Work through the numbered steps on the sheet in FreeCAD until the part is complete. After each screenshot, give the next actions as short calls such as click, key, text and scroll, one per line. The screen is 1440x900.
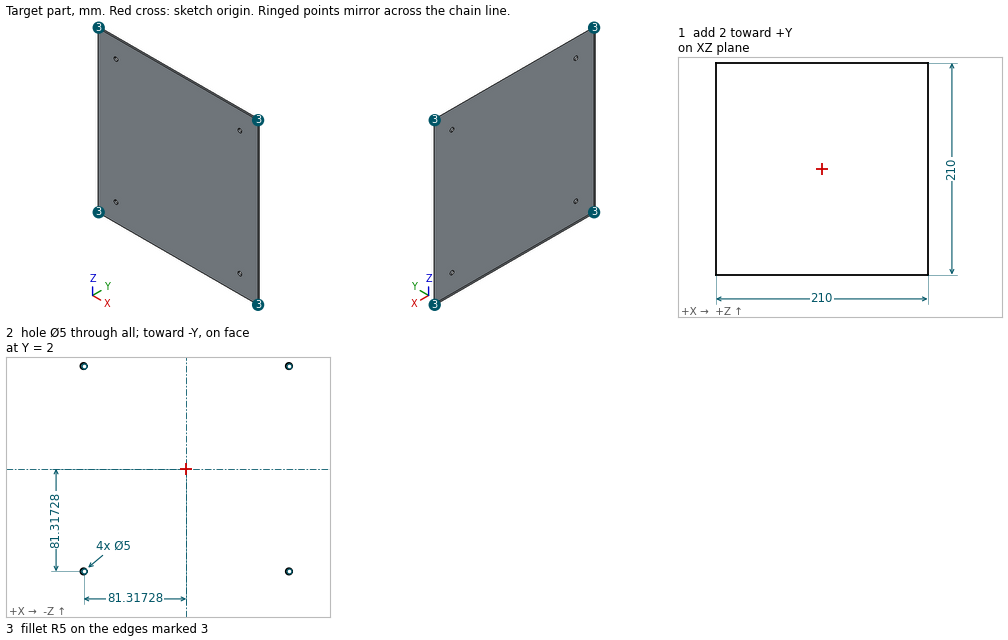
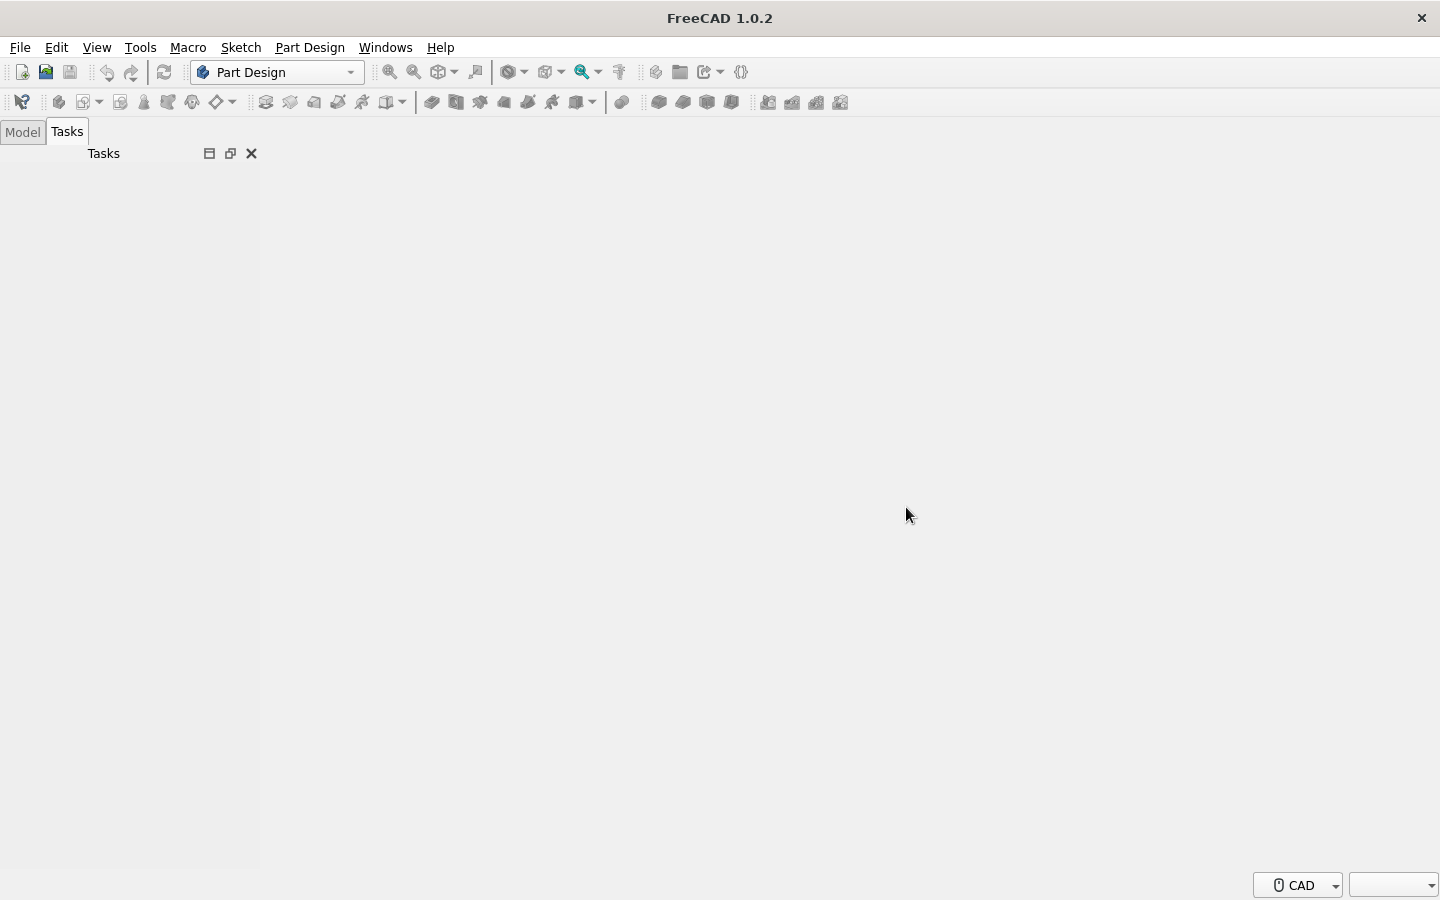
click(22, 72)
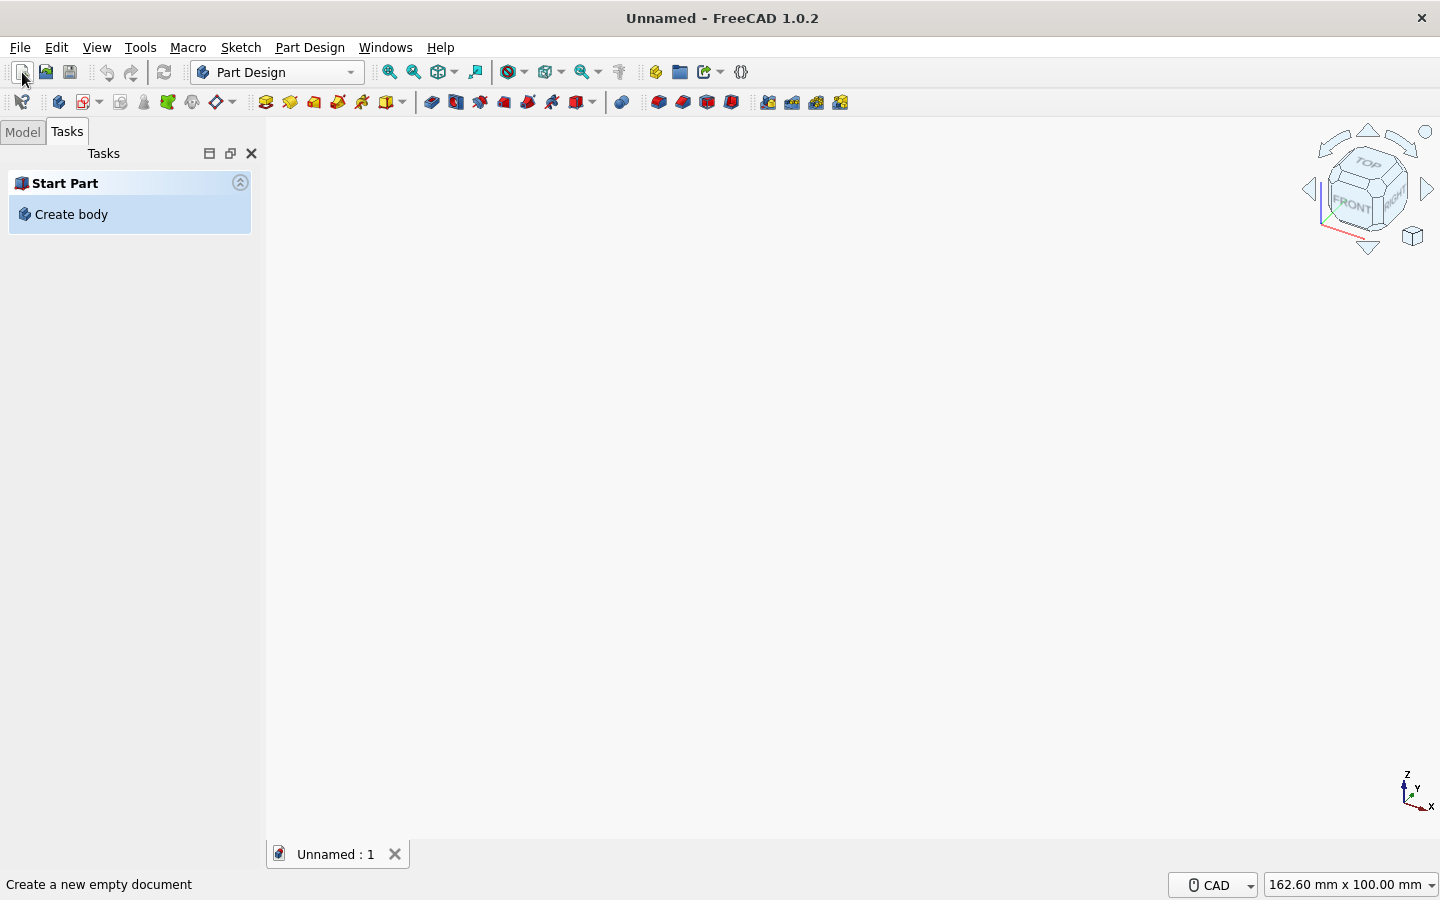
click(84, 102)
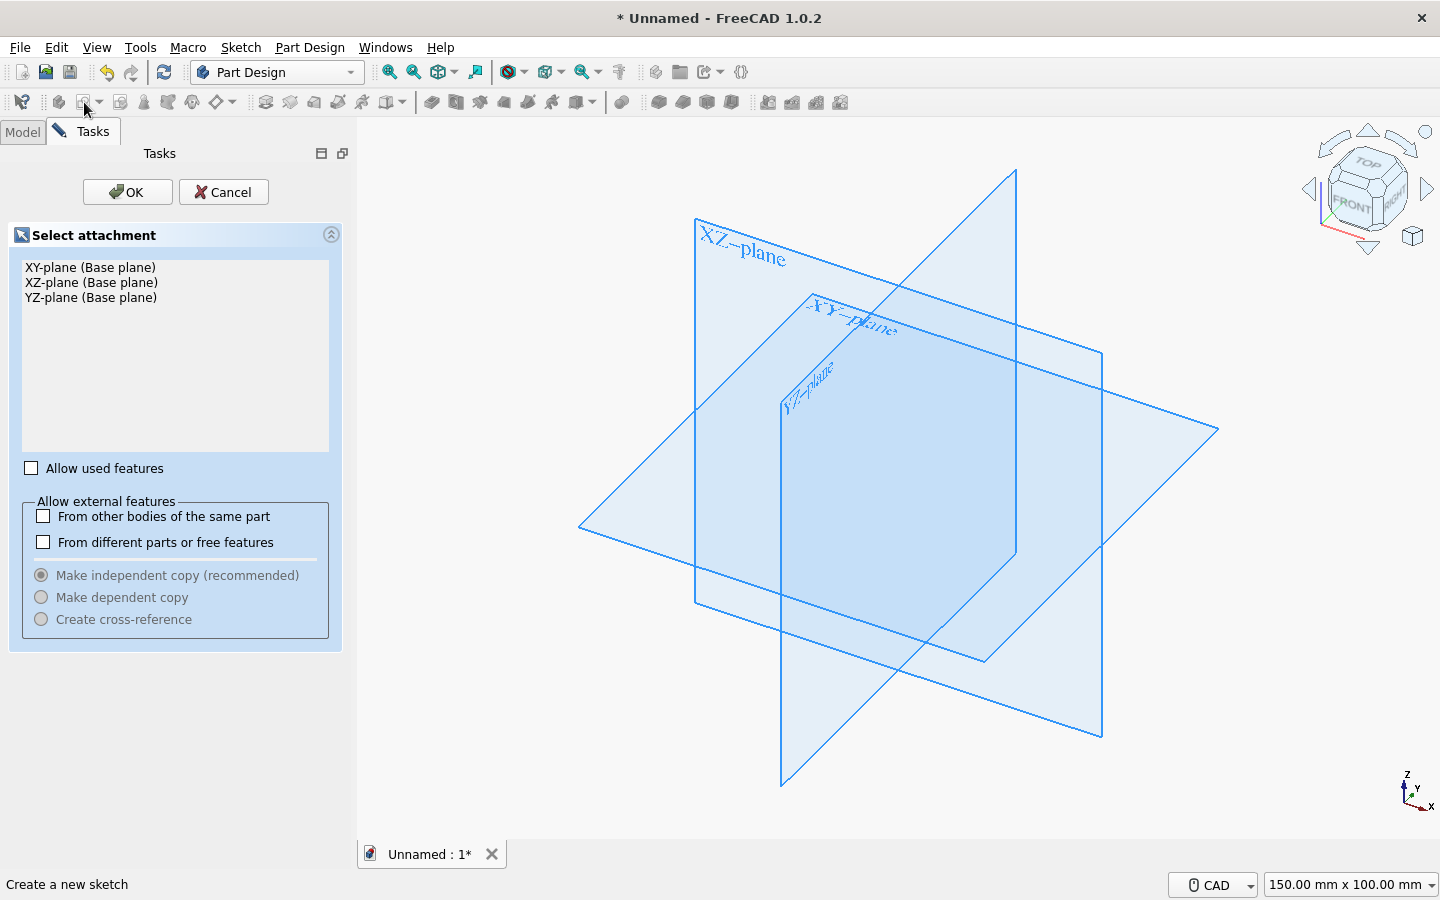
click(82, 282)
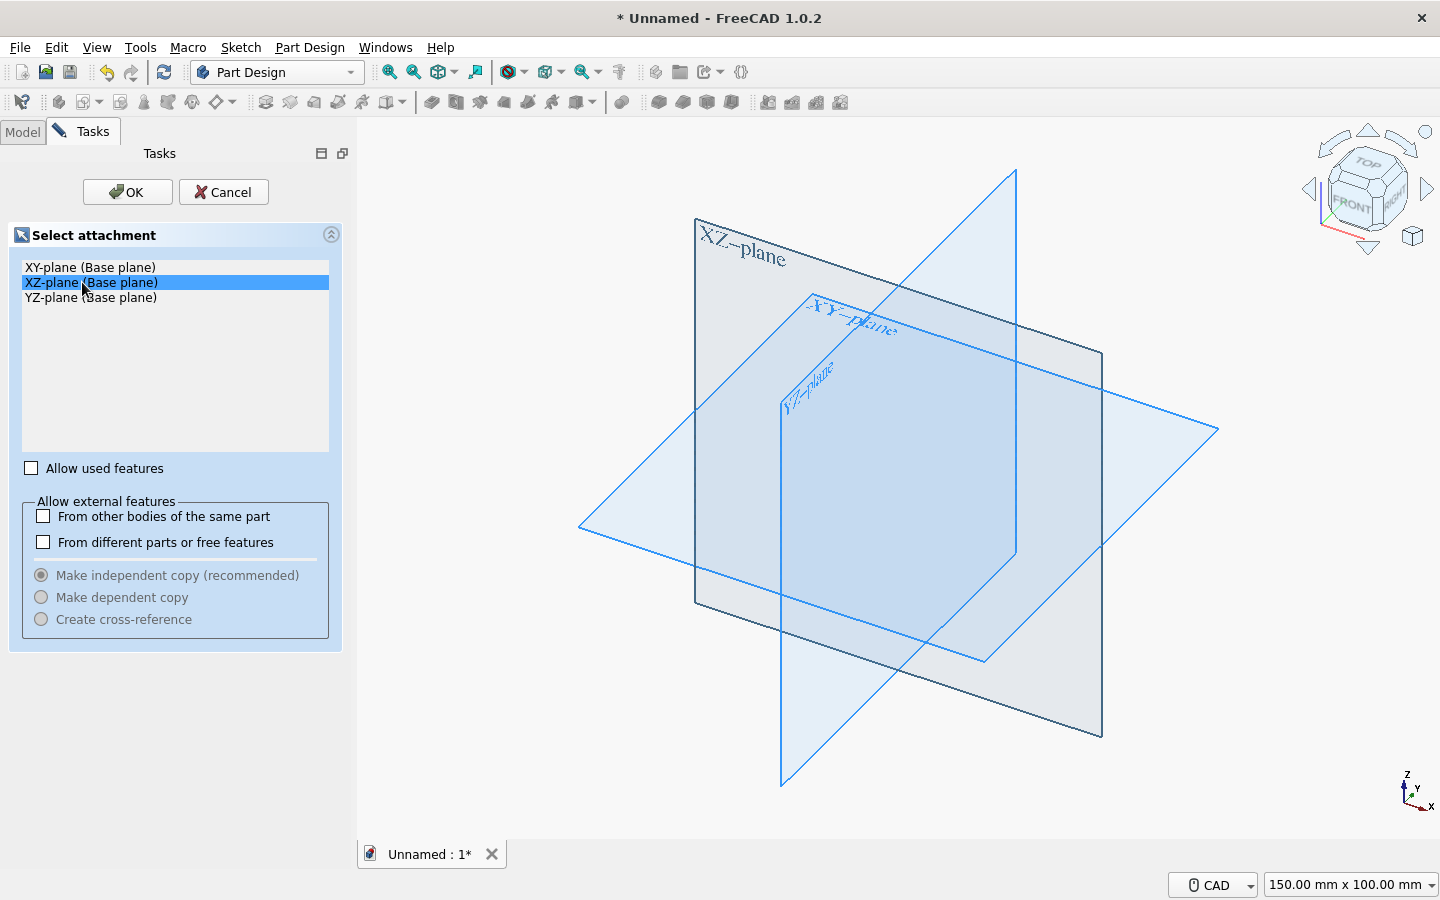
click(128, 192)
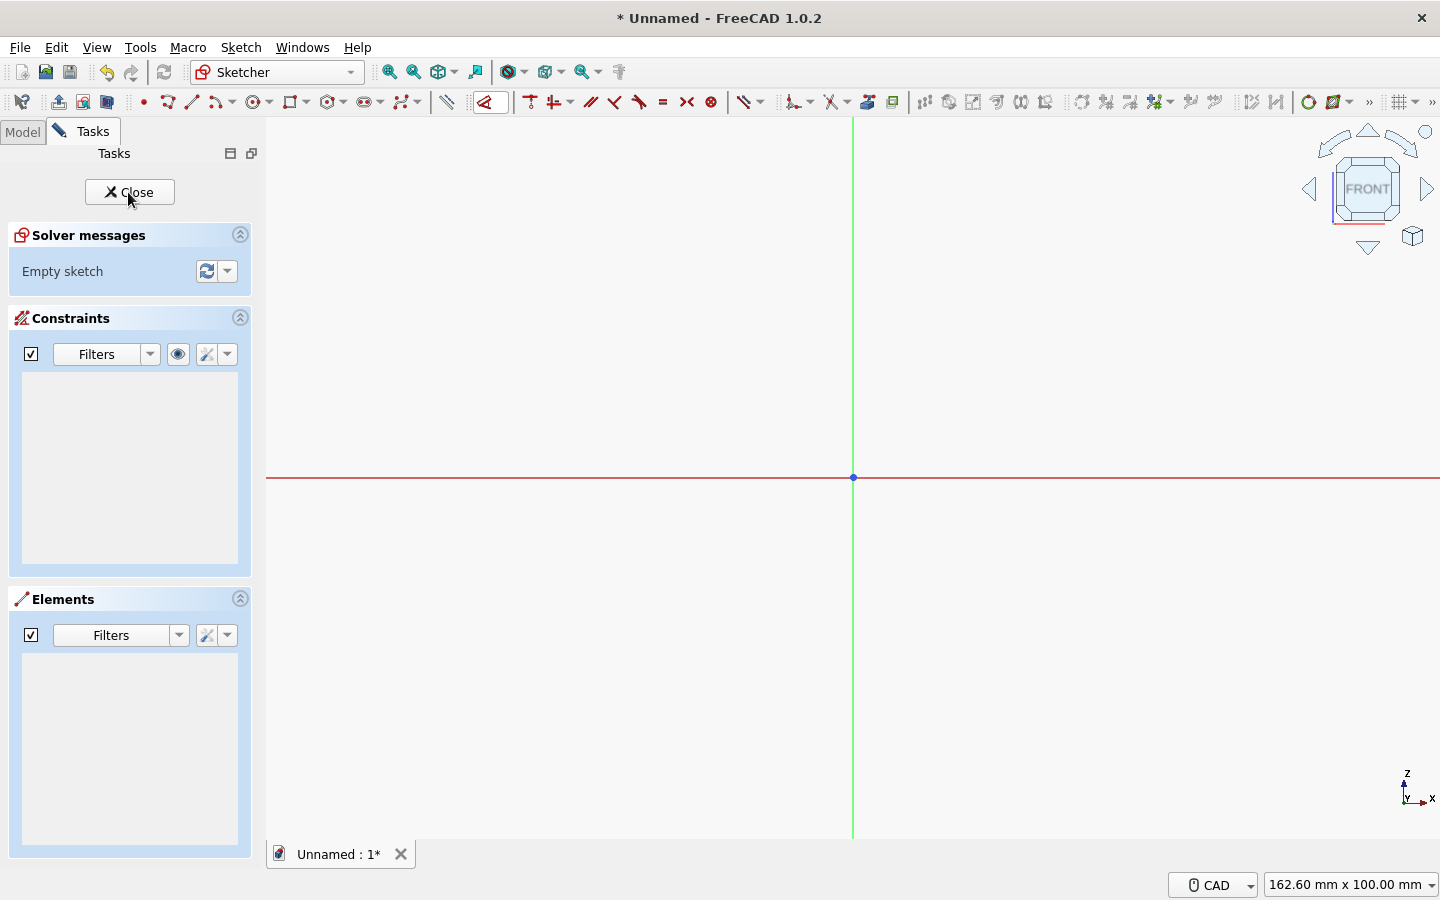
scroll(755, 478, down, 6)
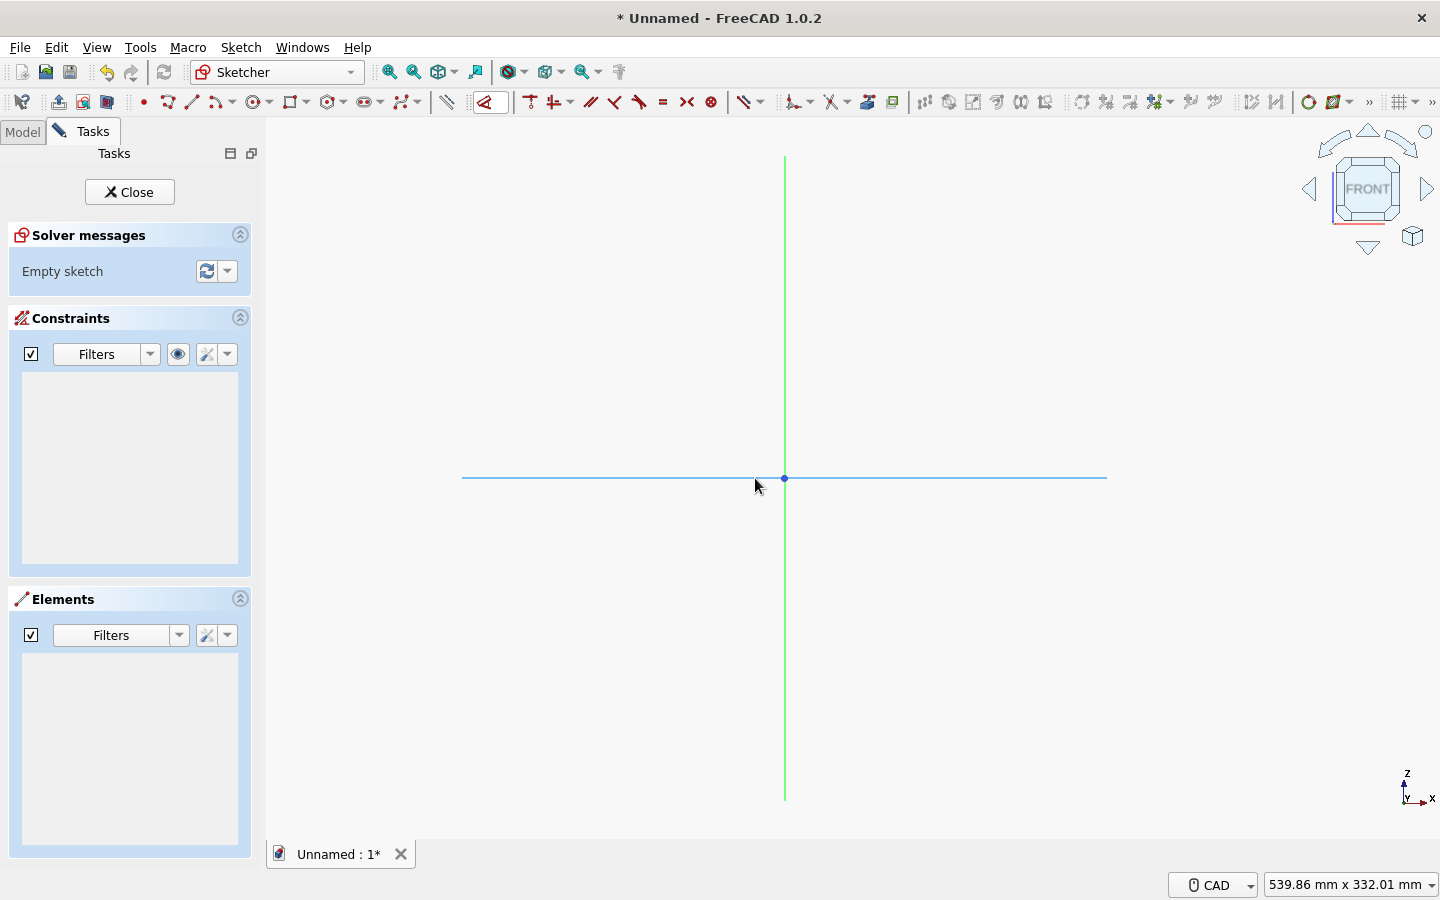
key(g)
key(v)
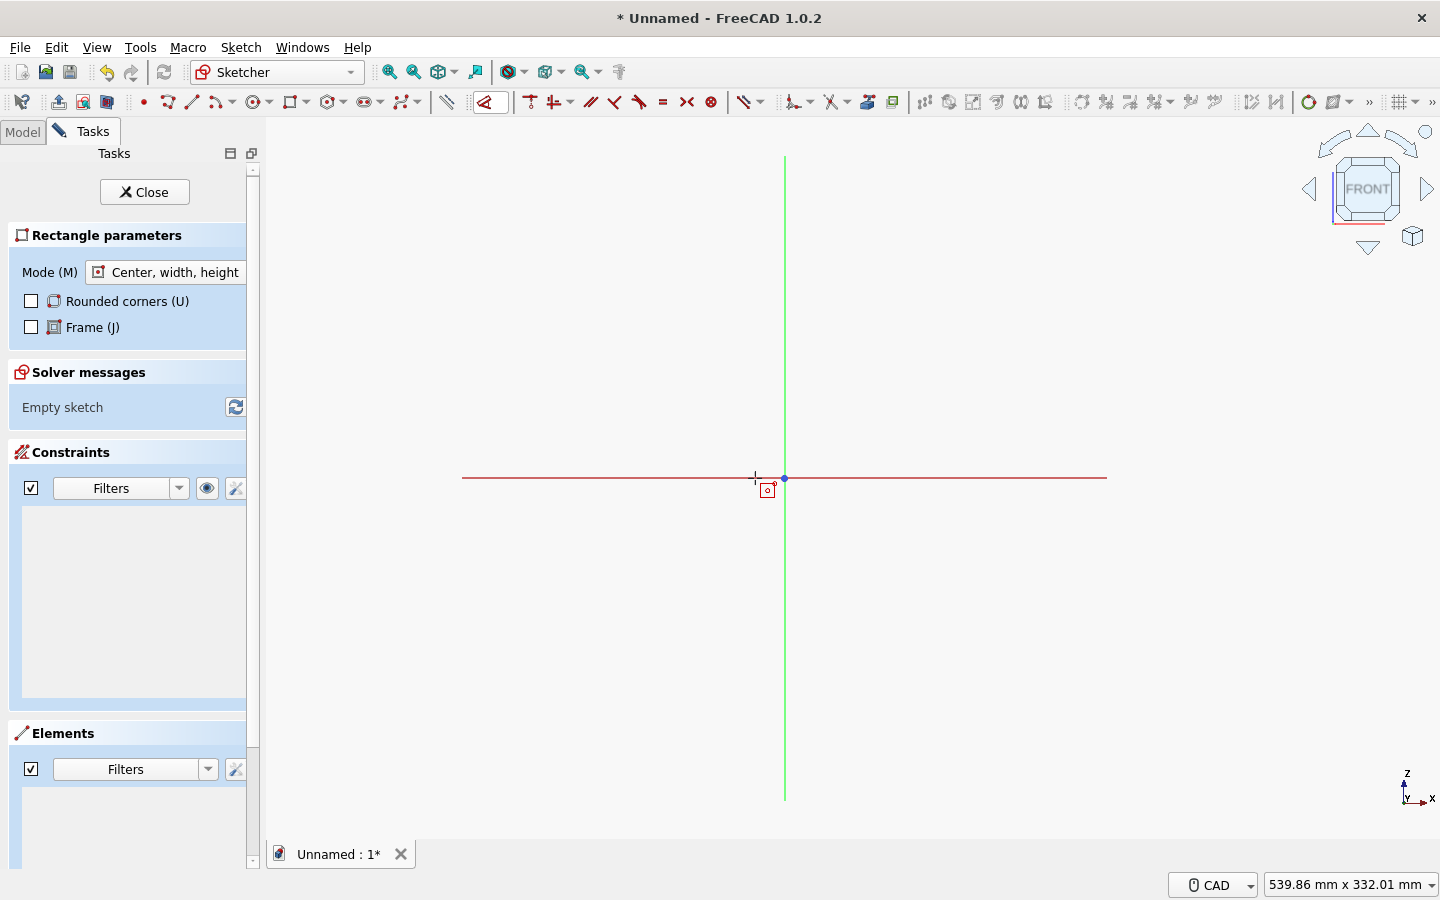
click(785, 478)
move(1013, 250)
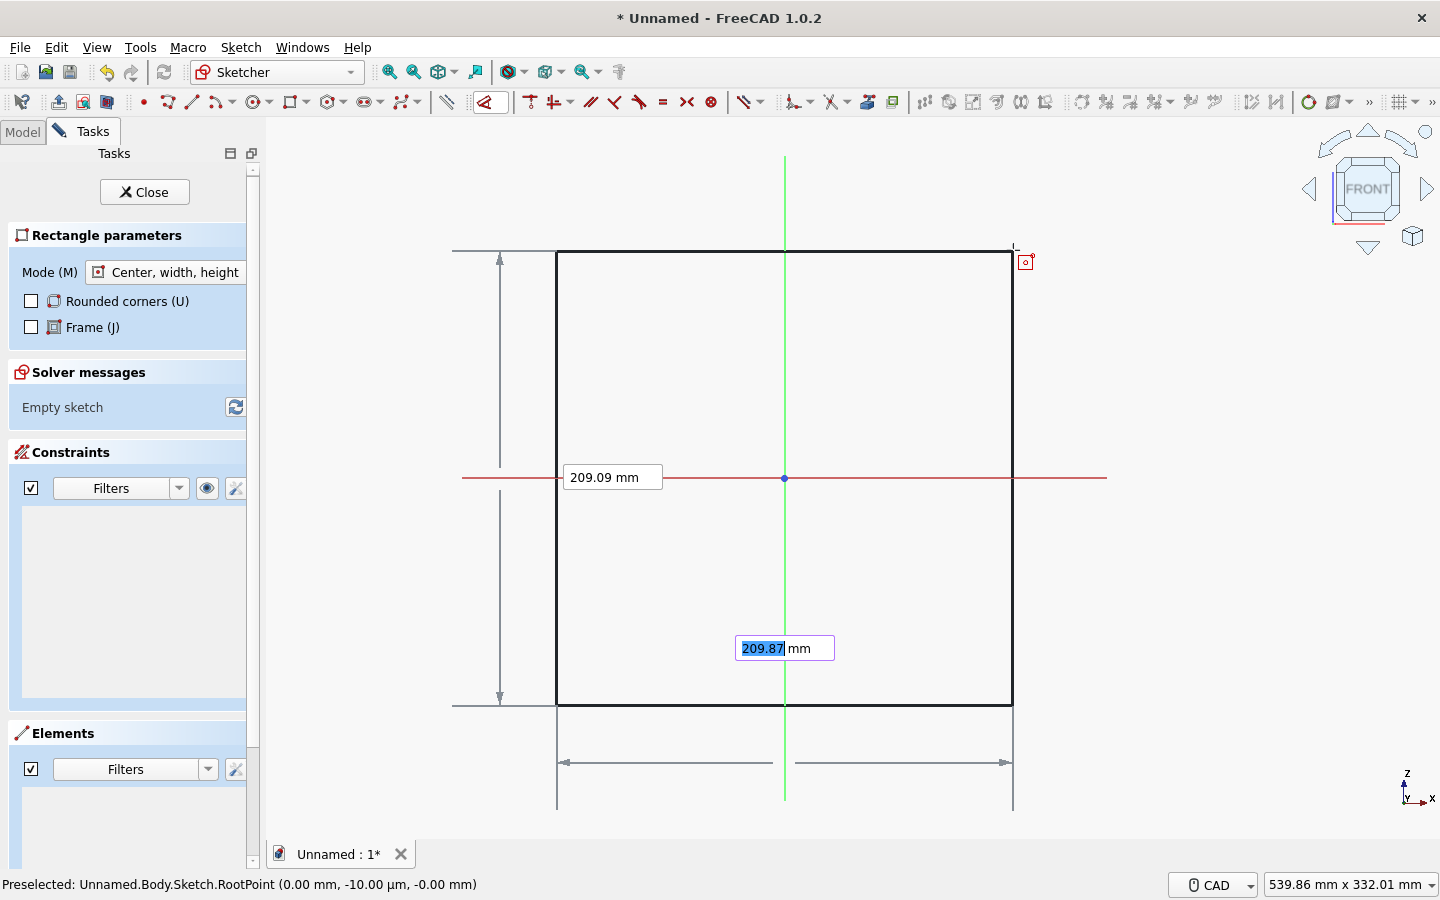
text(210)
key(Tab)
text(210)
key(Return)
key(Escape)